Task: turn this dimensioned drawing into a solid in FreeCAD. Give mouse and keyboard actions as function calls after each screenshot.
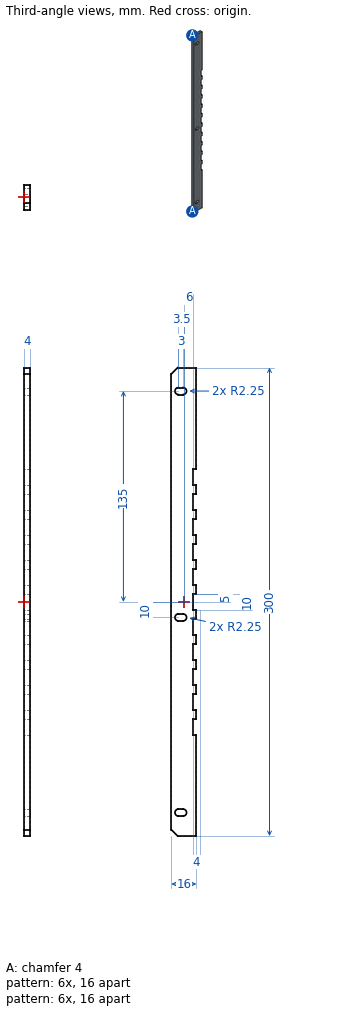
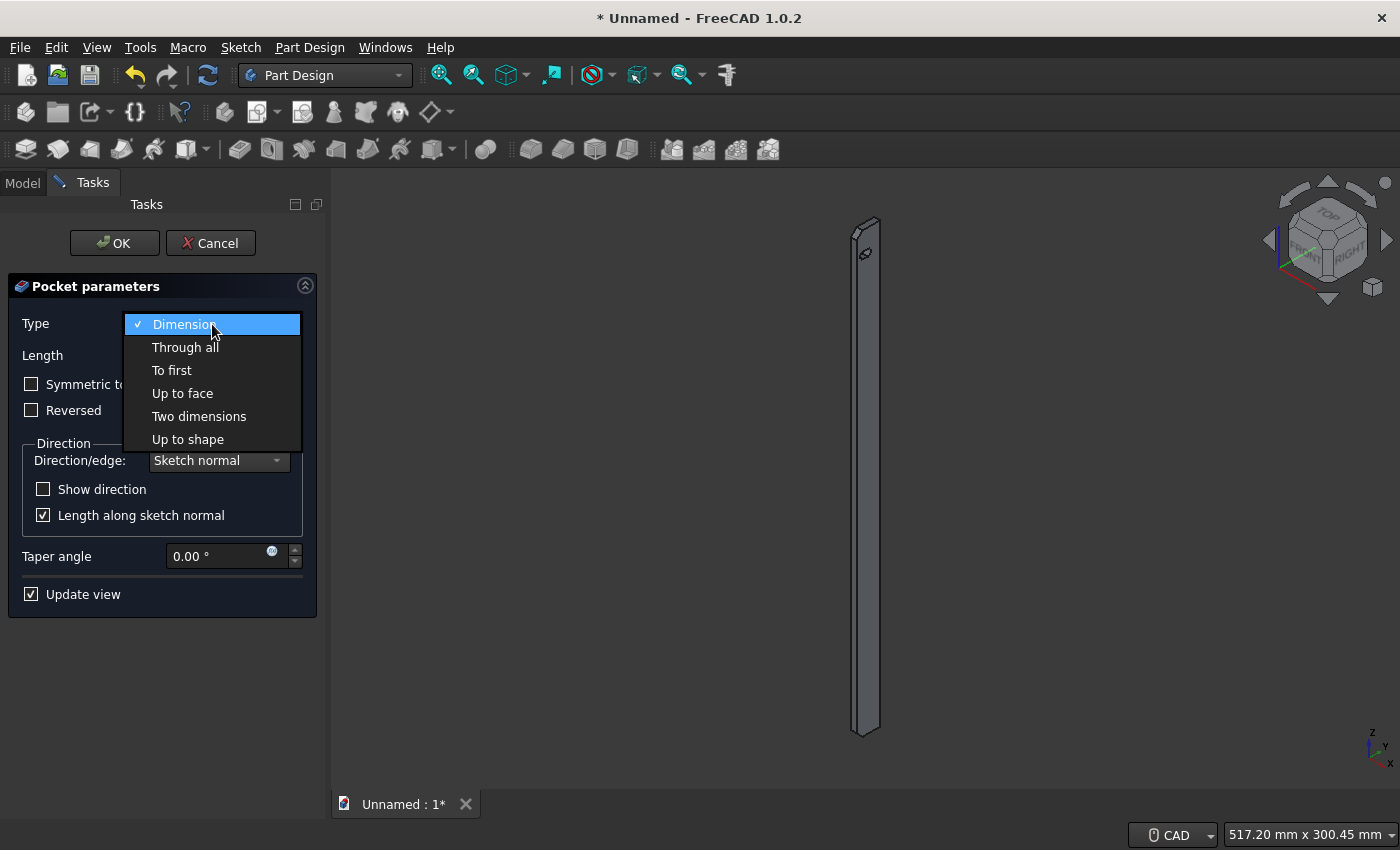
click(212, 348)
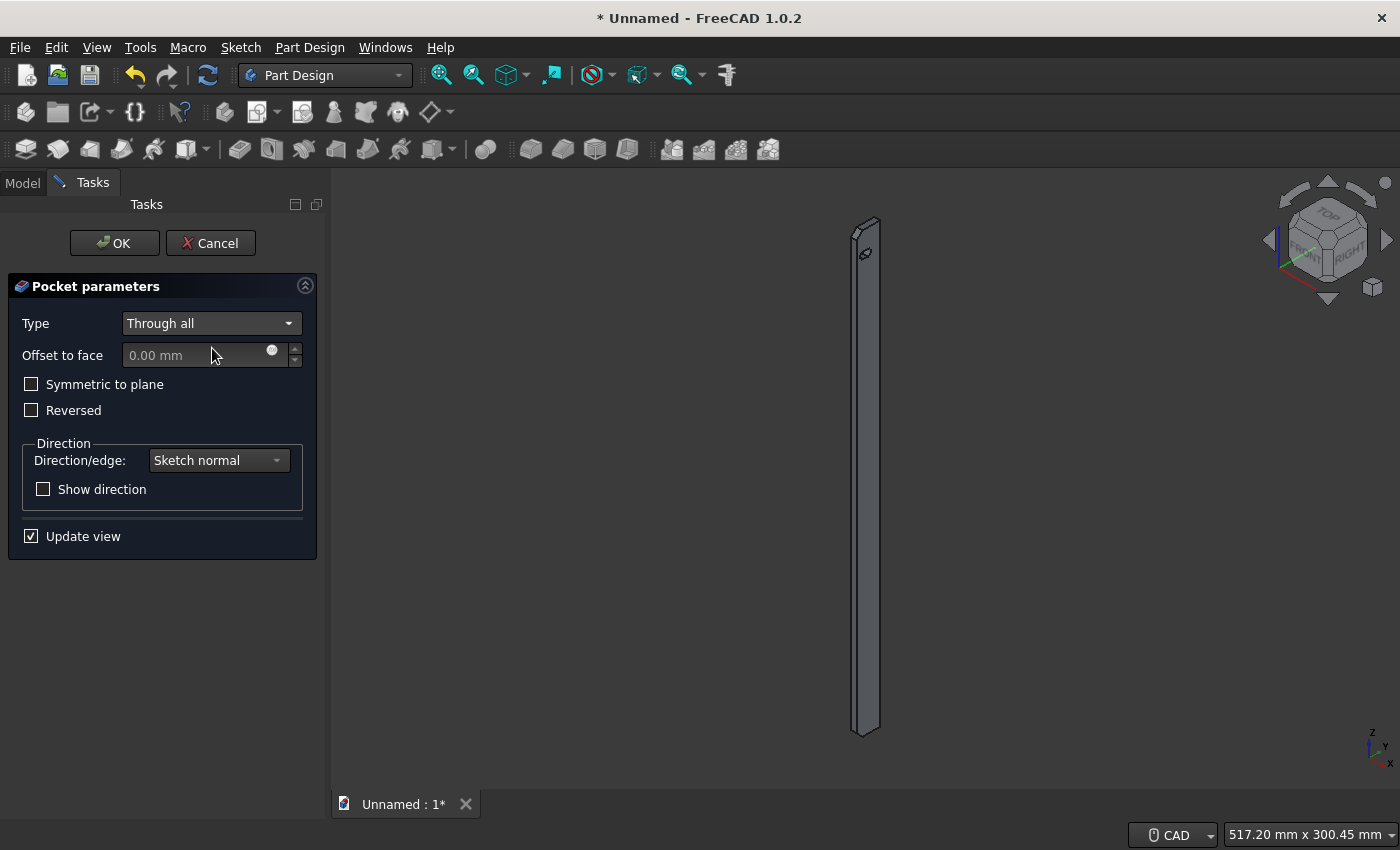
click(115, 243)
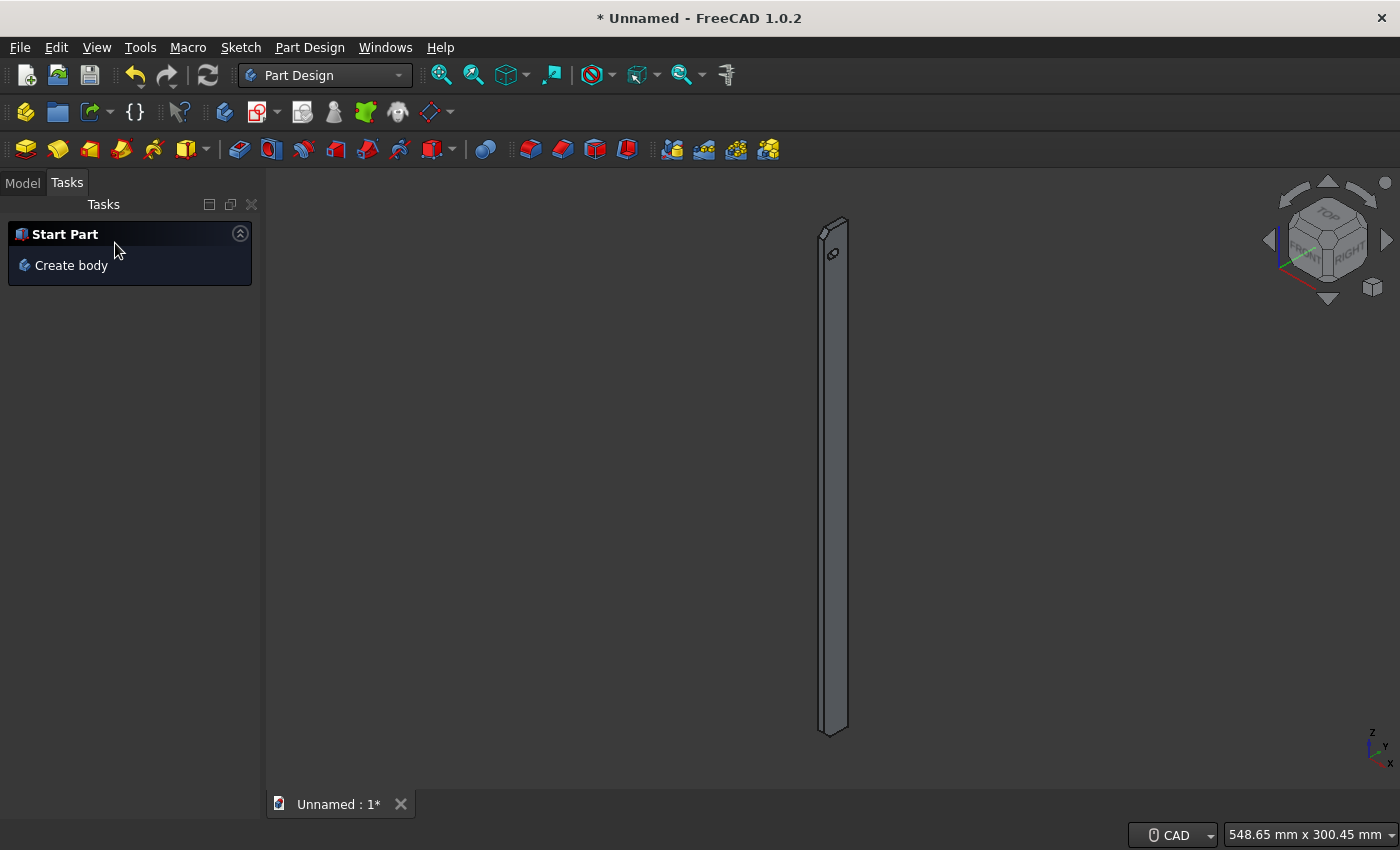
click(23, 182)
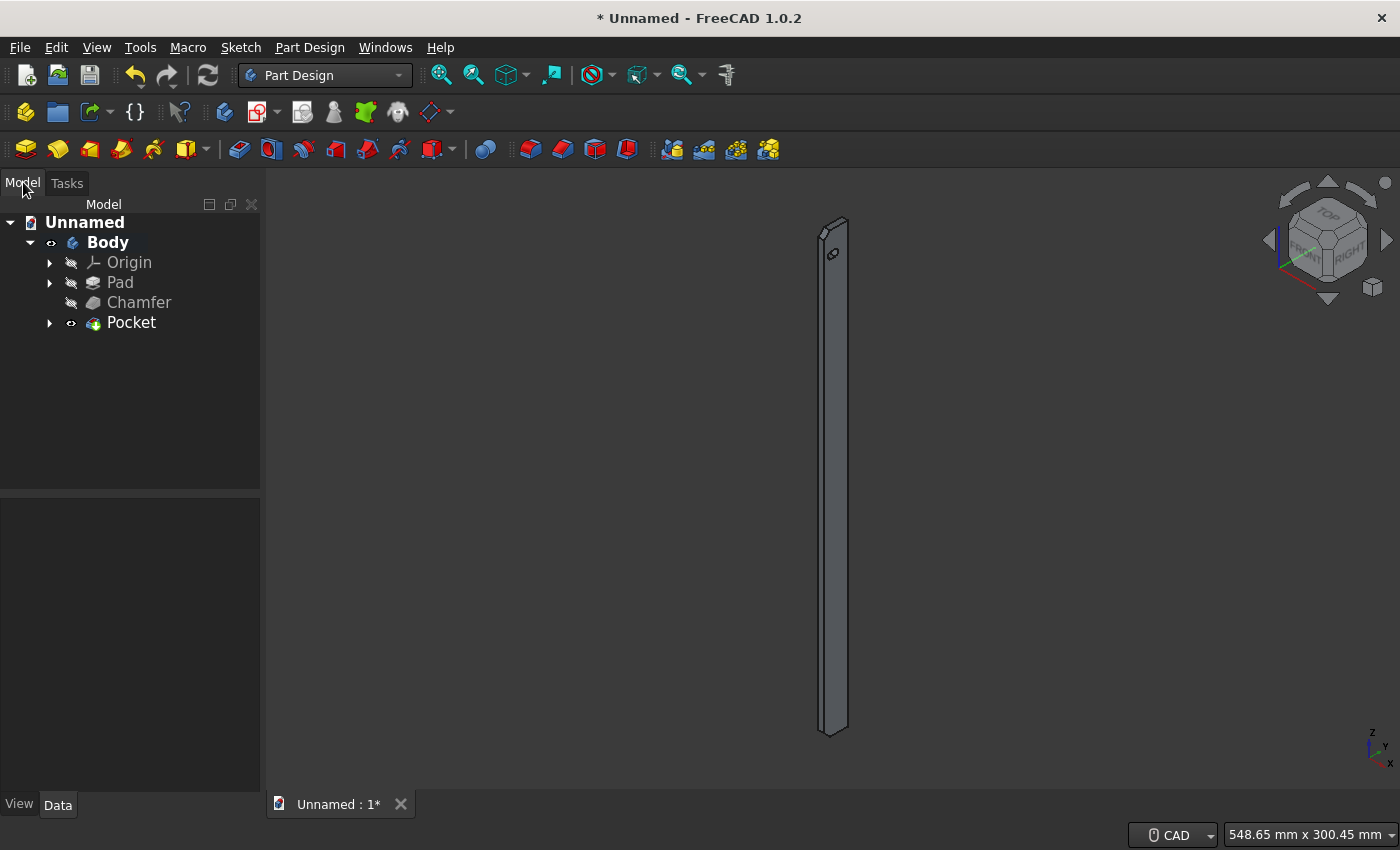
click(116, 323)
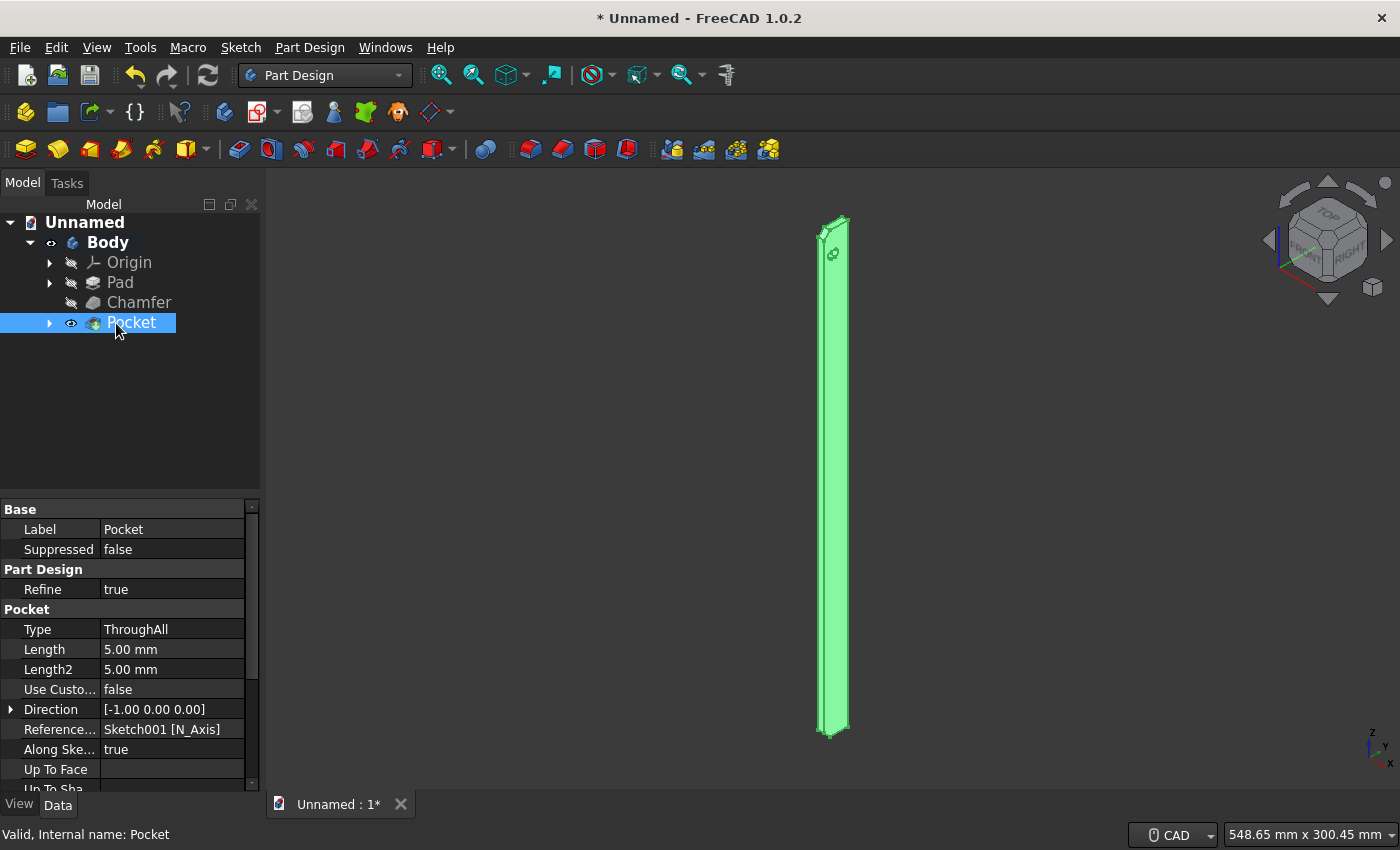
click(672, 150)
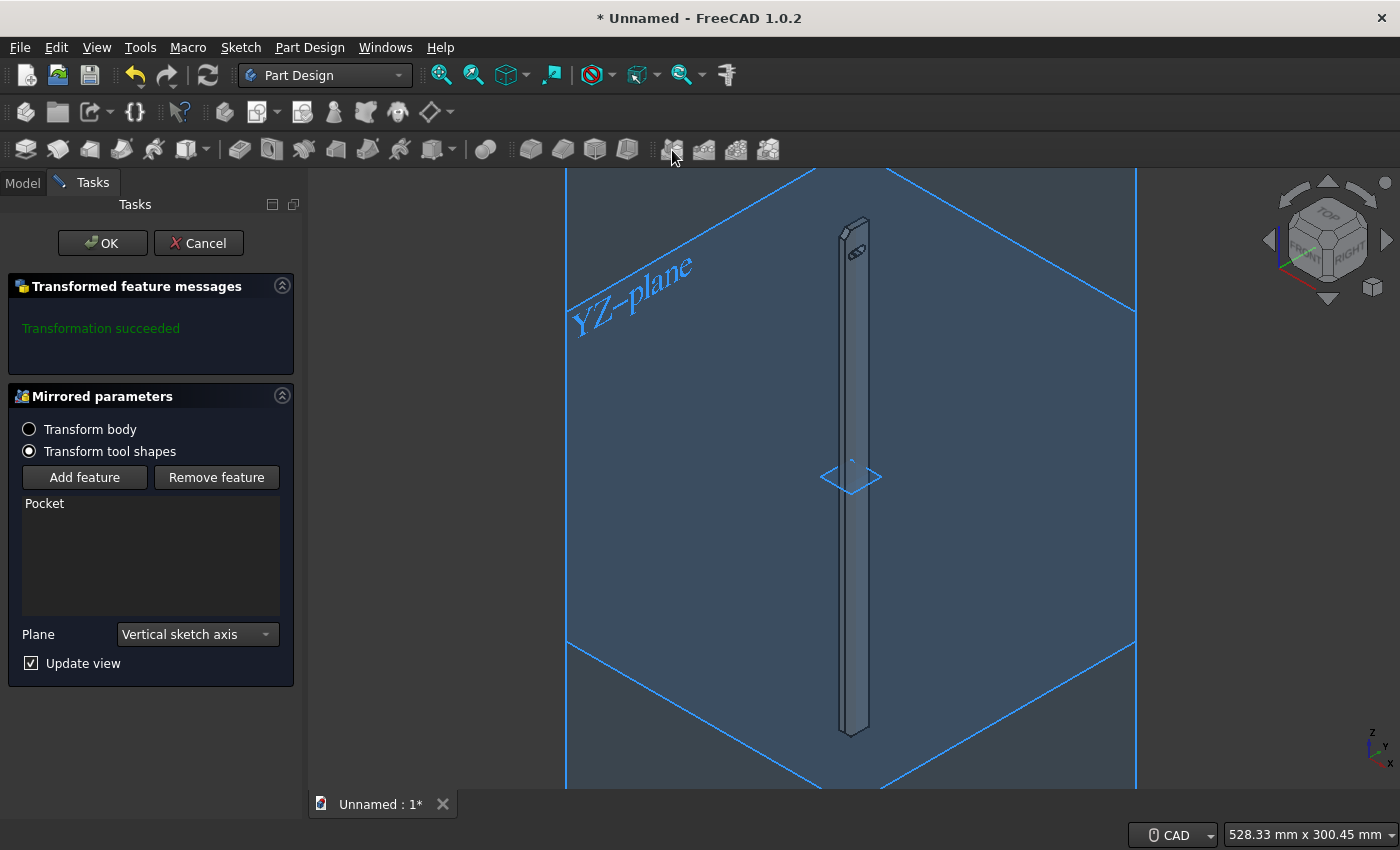
click(198, 634)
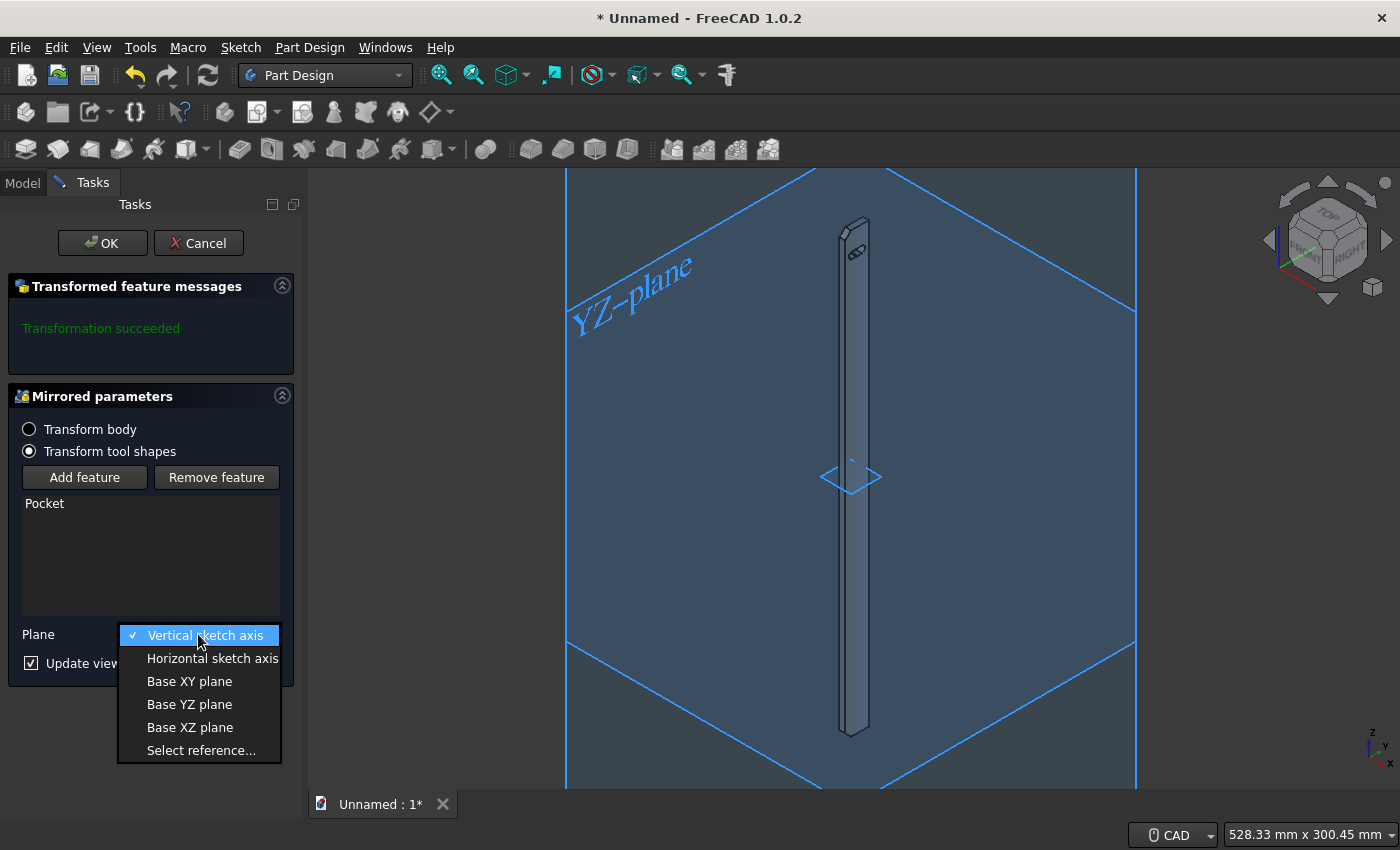
click(198, 682)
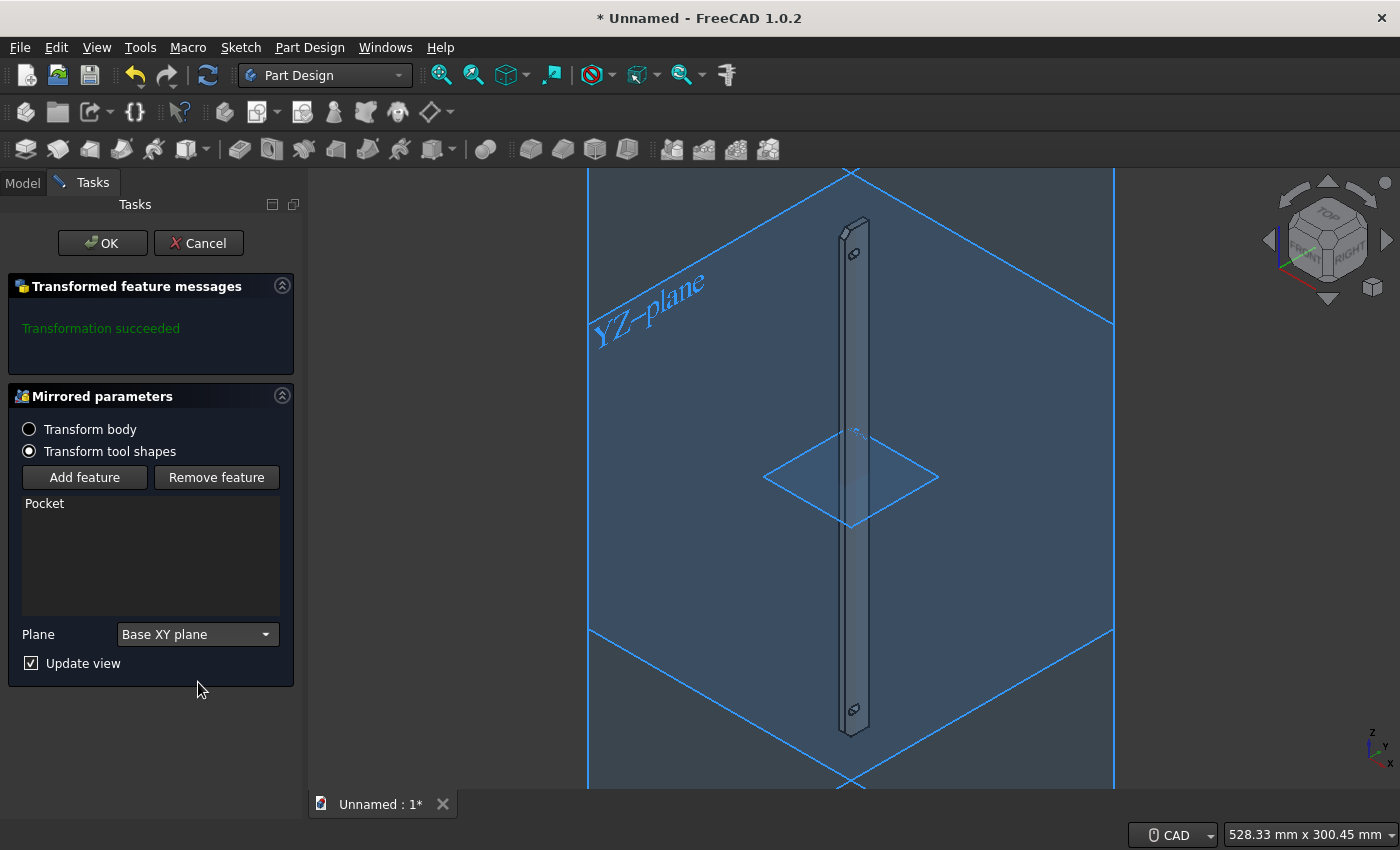
click(103, 243)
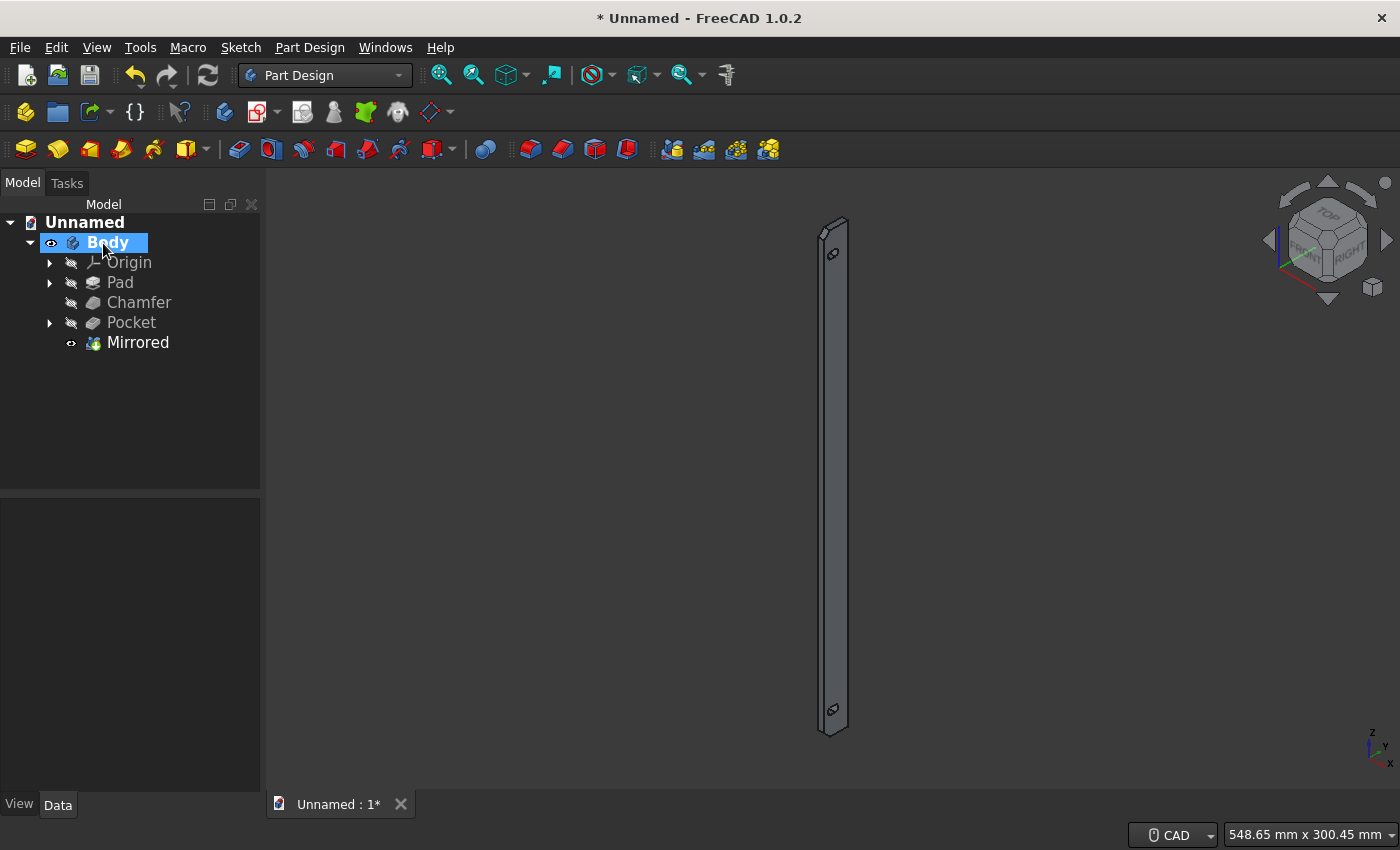
click(836, 479)